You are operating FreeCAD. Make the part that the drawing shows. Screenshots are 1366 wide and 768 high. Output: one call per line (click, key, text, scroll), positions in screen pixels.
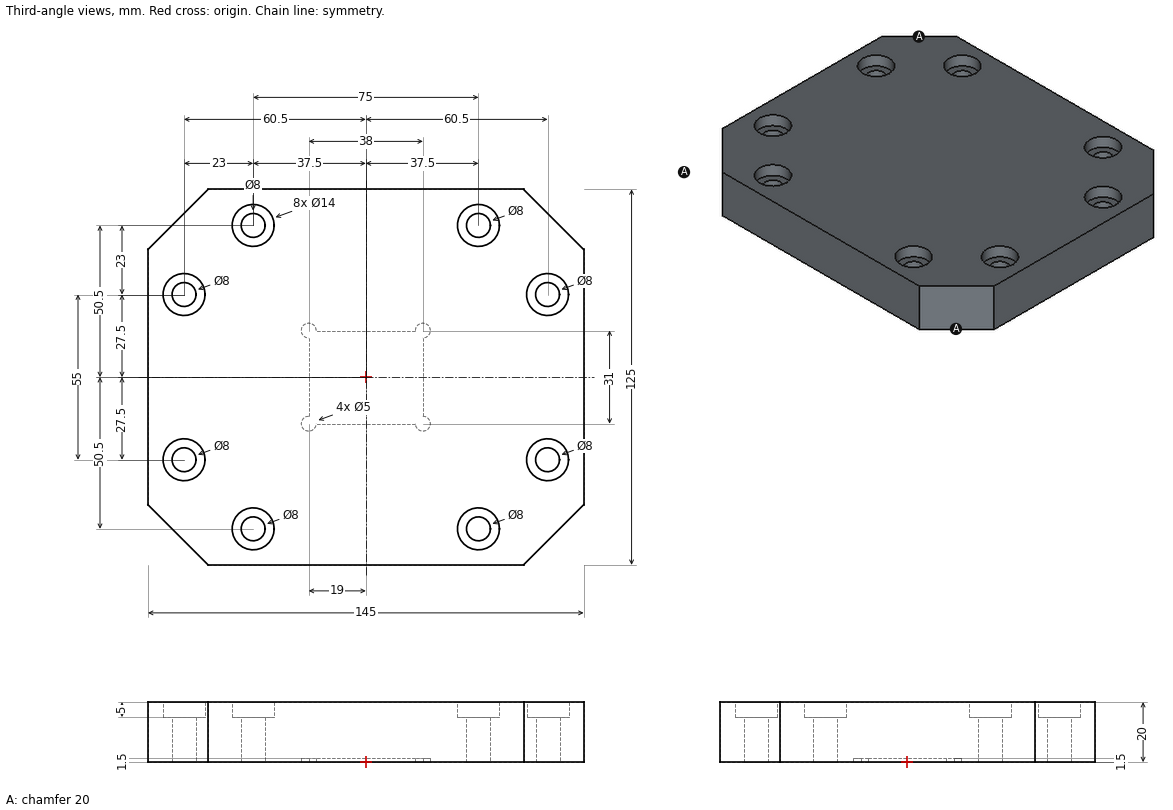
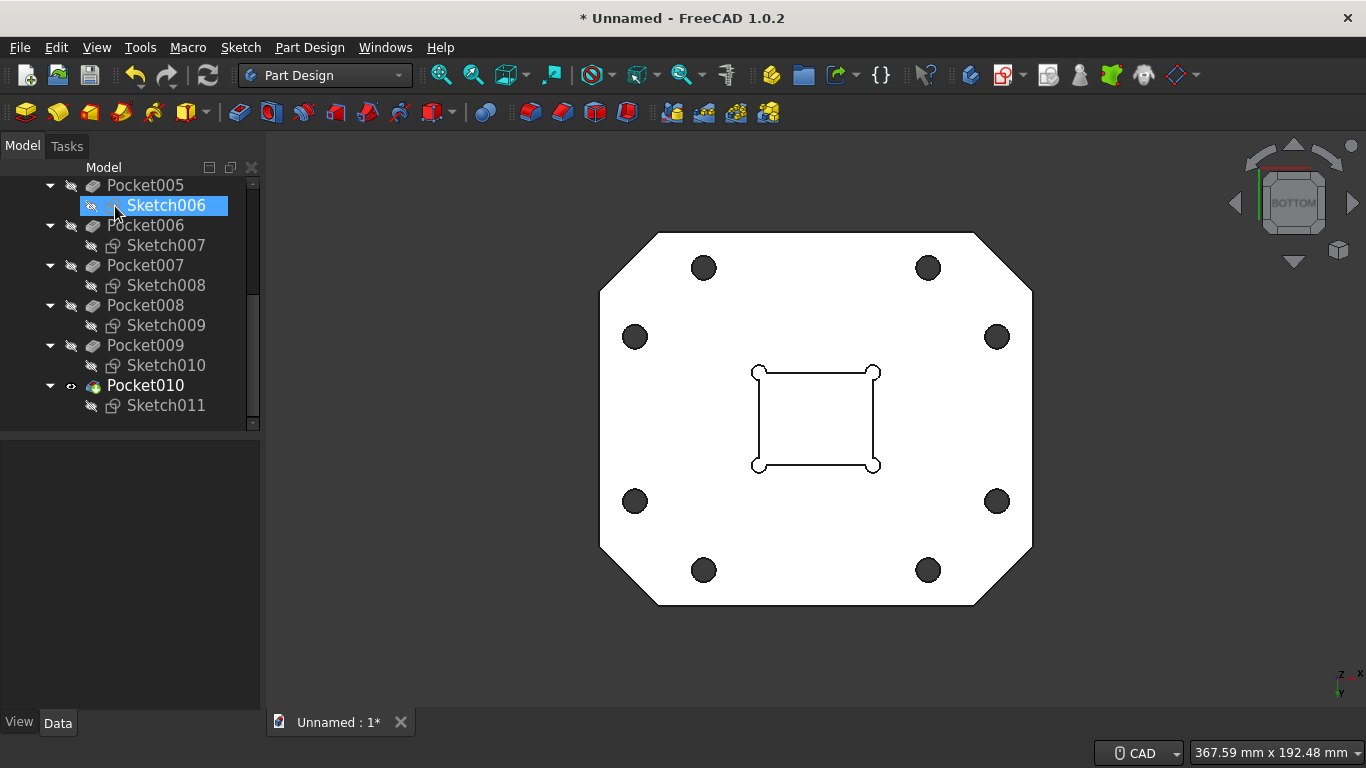
key(0)